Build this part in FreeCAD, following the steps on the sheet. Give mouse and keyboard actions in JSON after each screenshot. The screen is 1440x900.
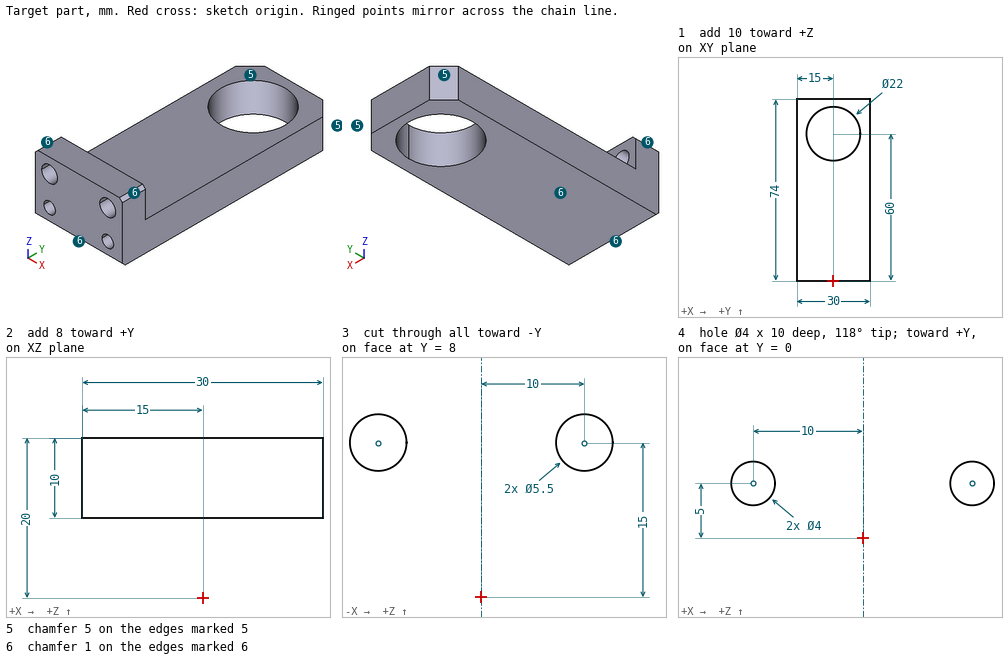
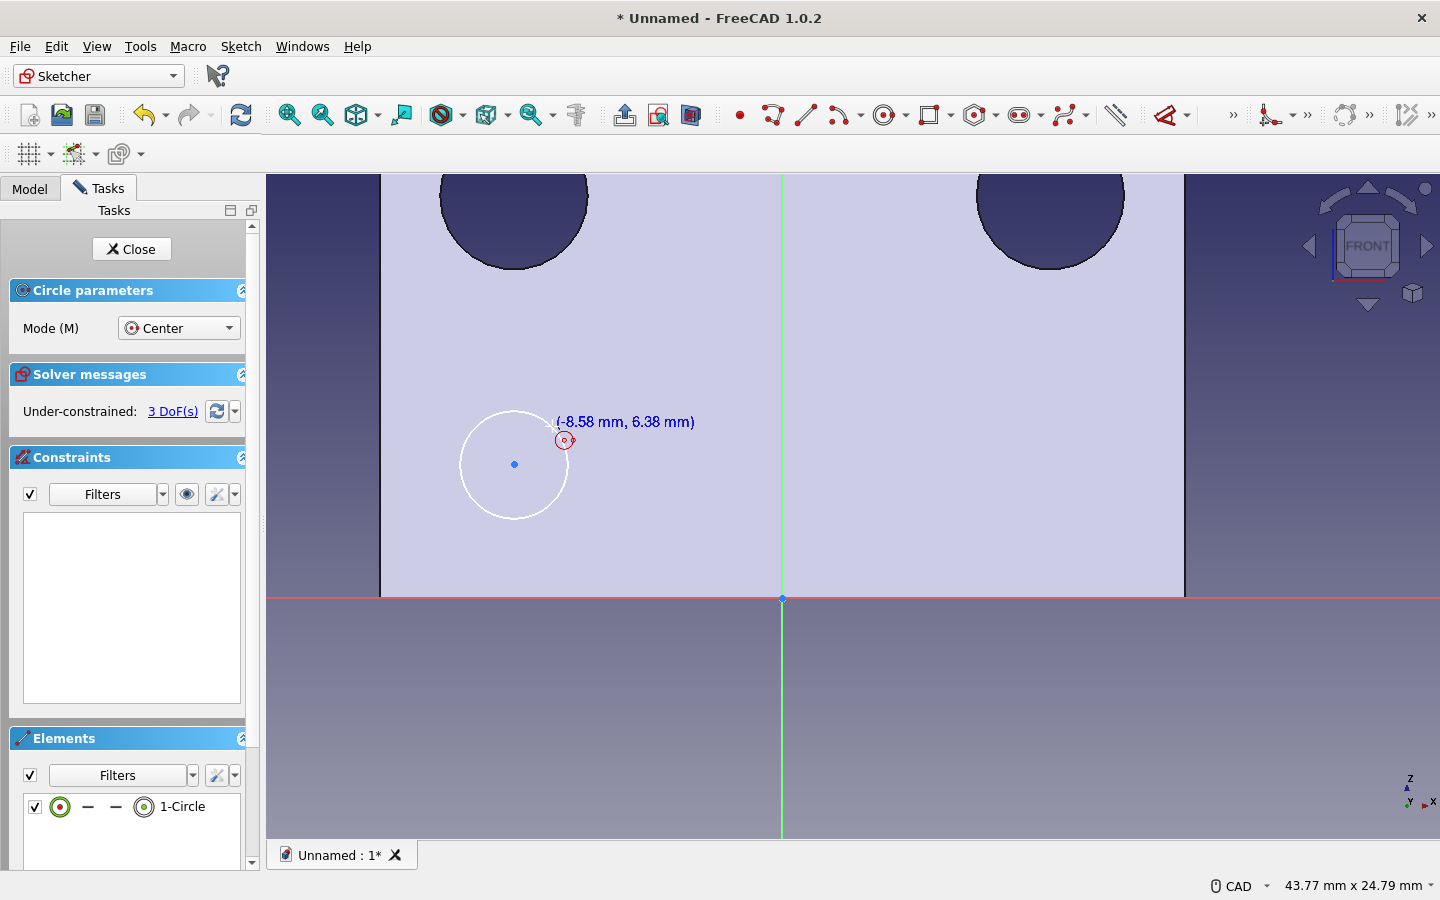
{"action": "left_click", "coordinate": [1050, 464]}
{"action": "left_click", "coordinate": [1088, 426]}
{"action": "key", "text": "Escape"}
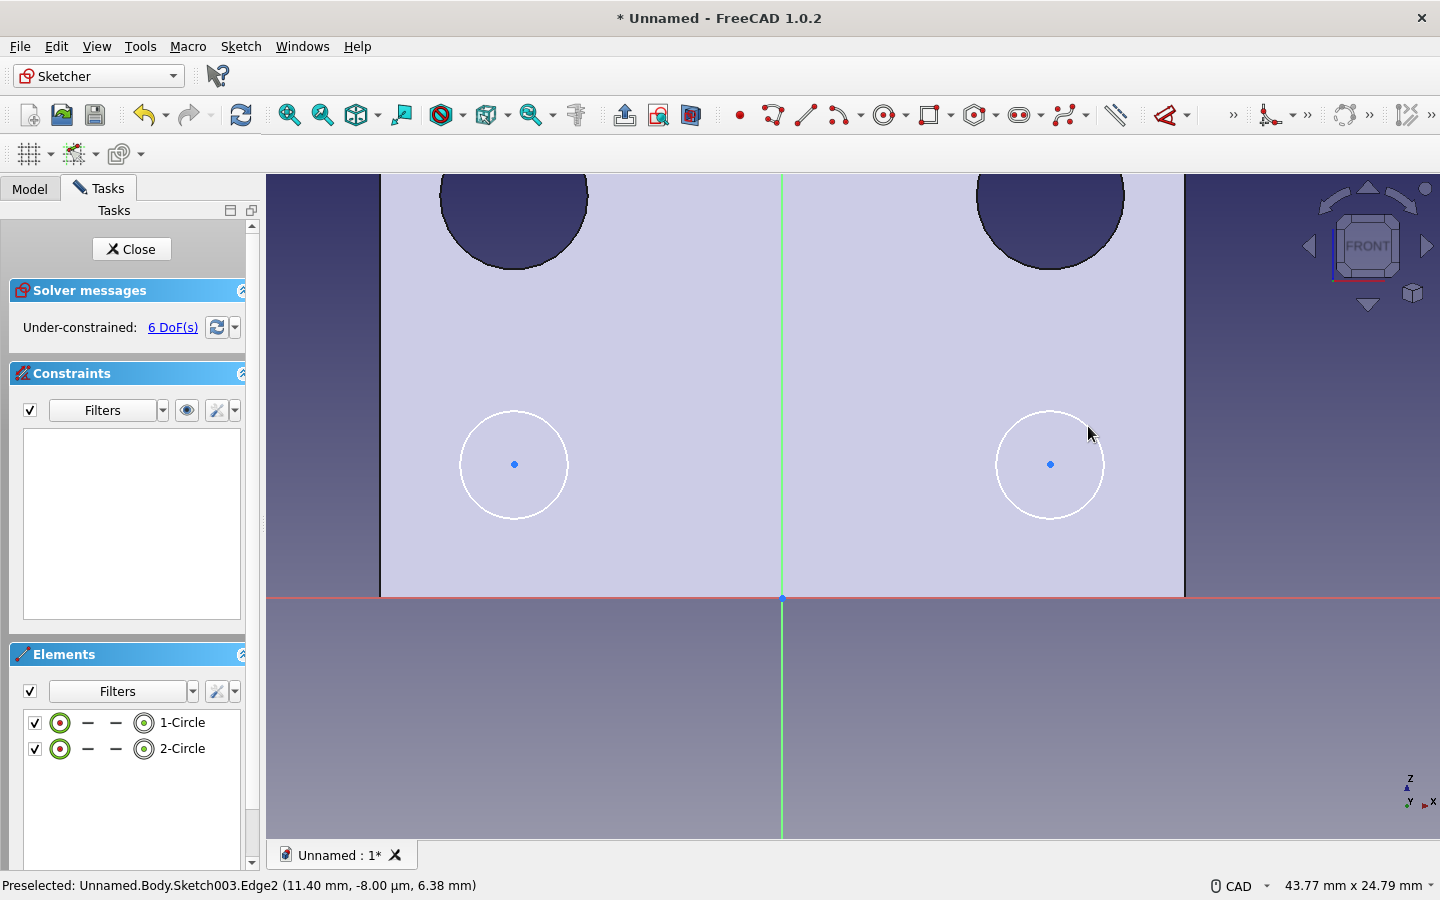
{"action": "left_click", "coordinate": [552, 427]}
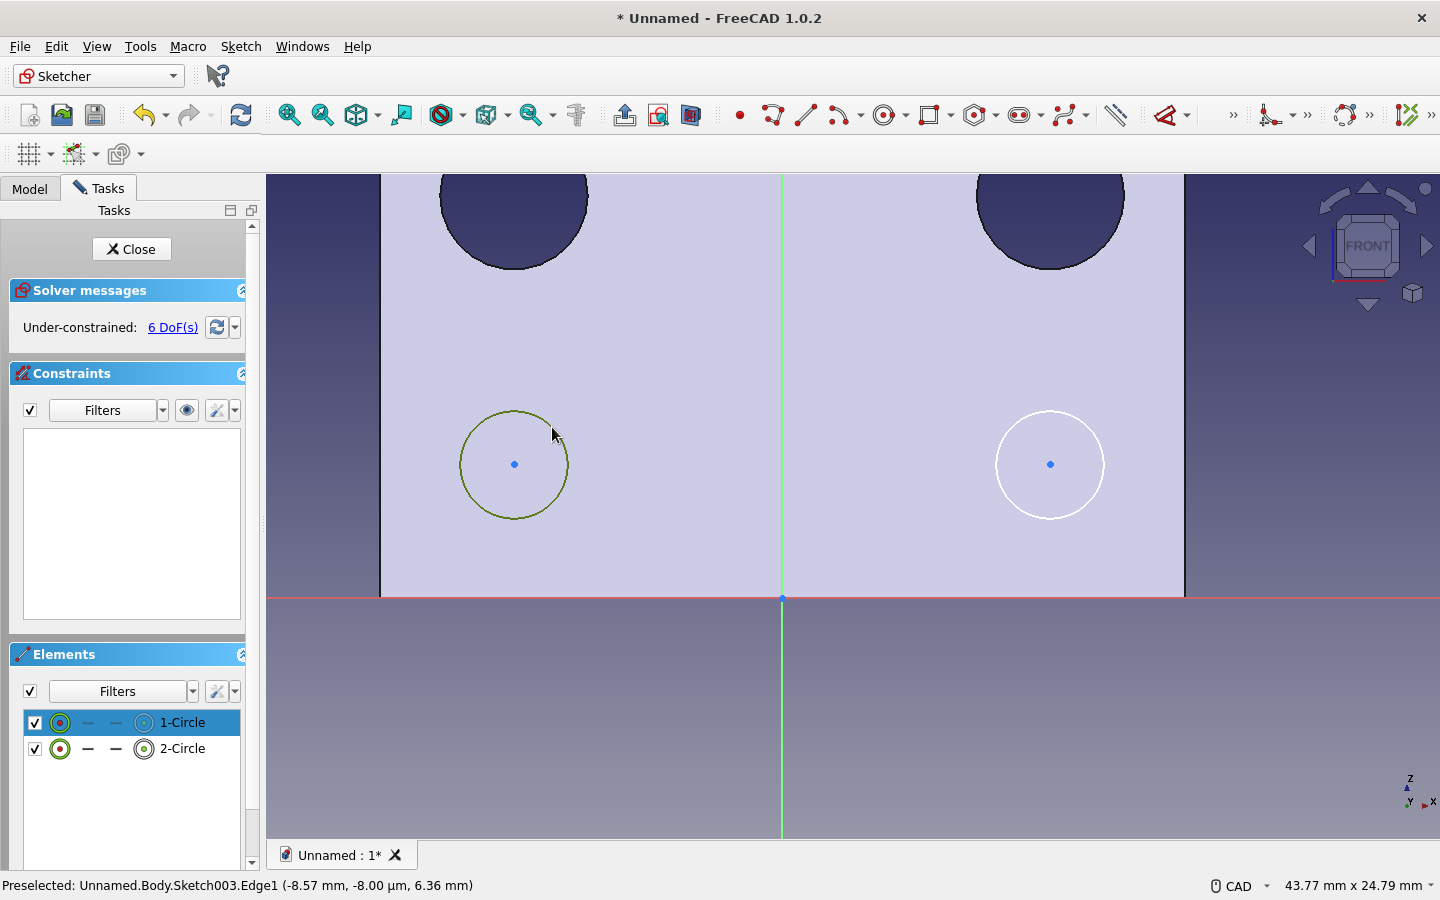
{"action": "left_click", "coordinate": [1088, 427]}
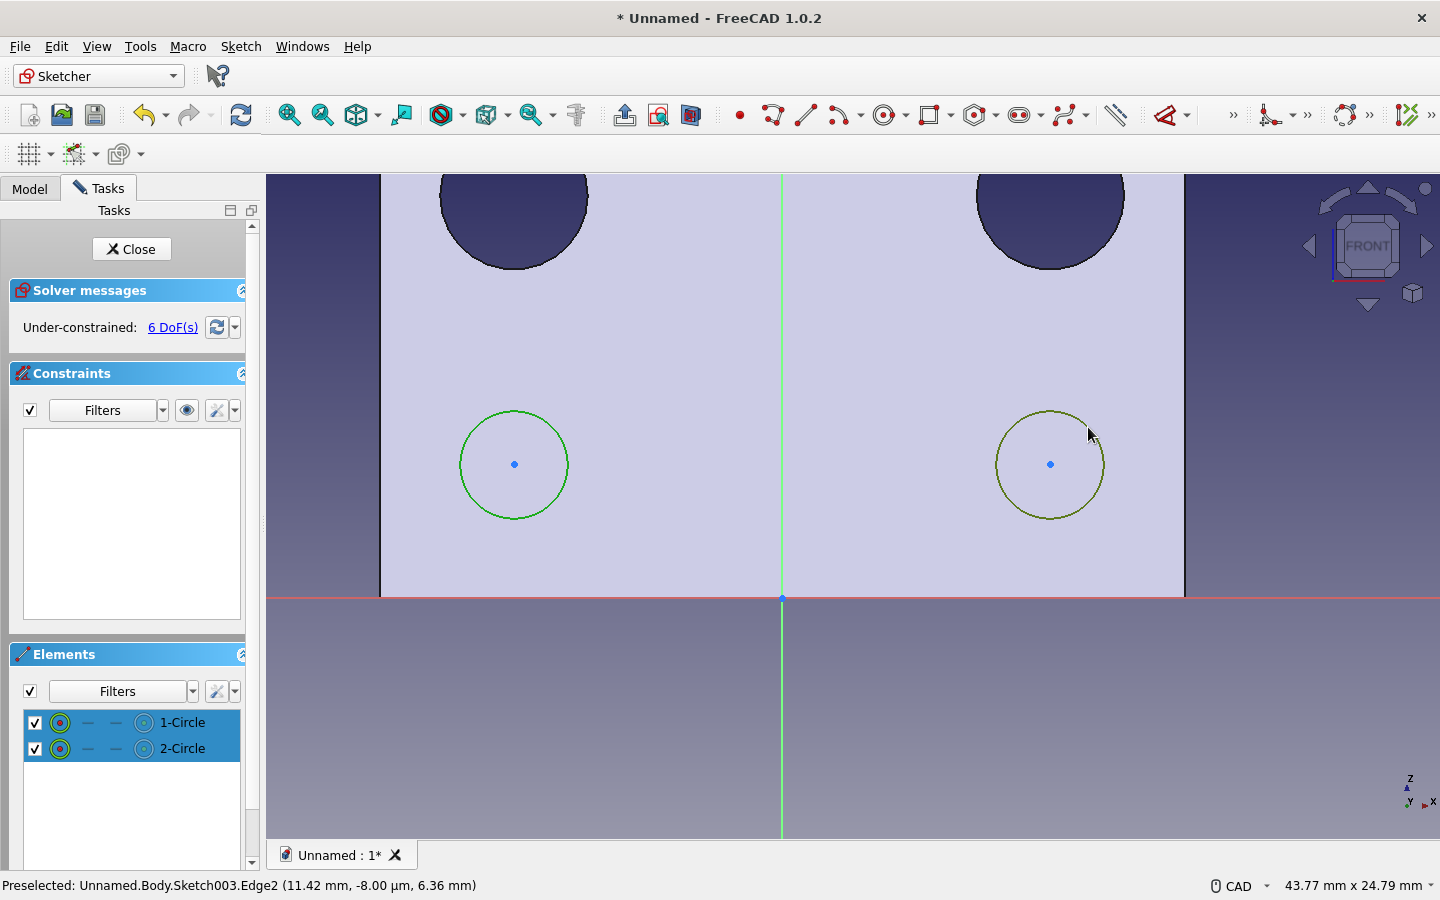
{"action": "key", "text": "e"}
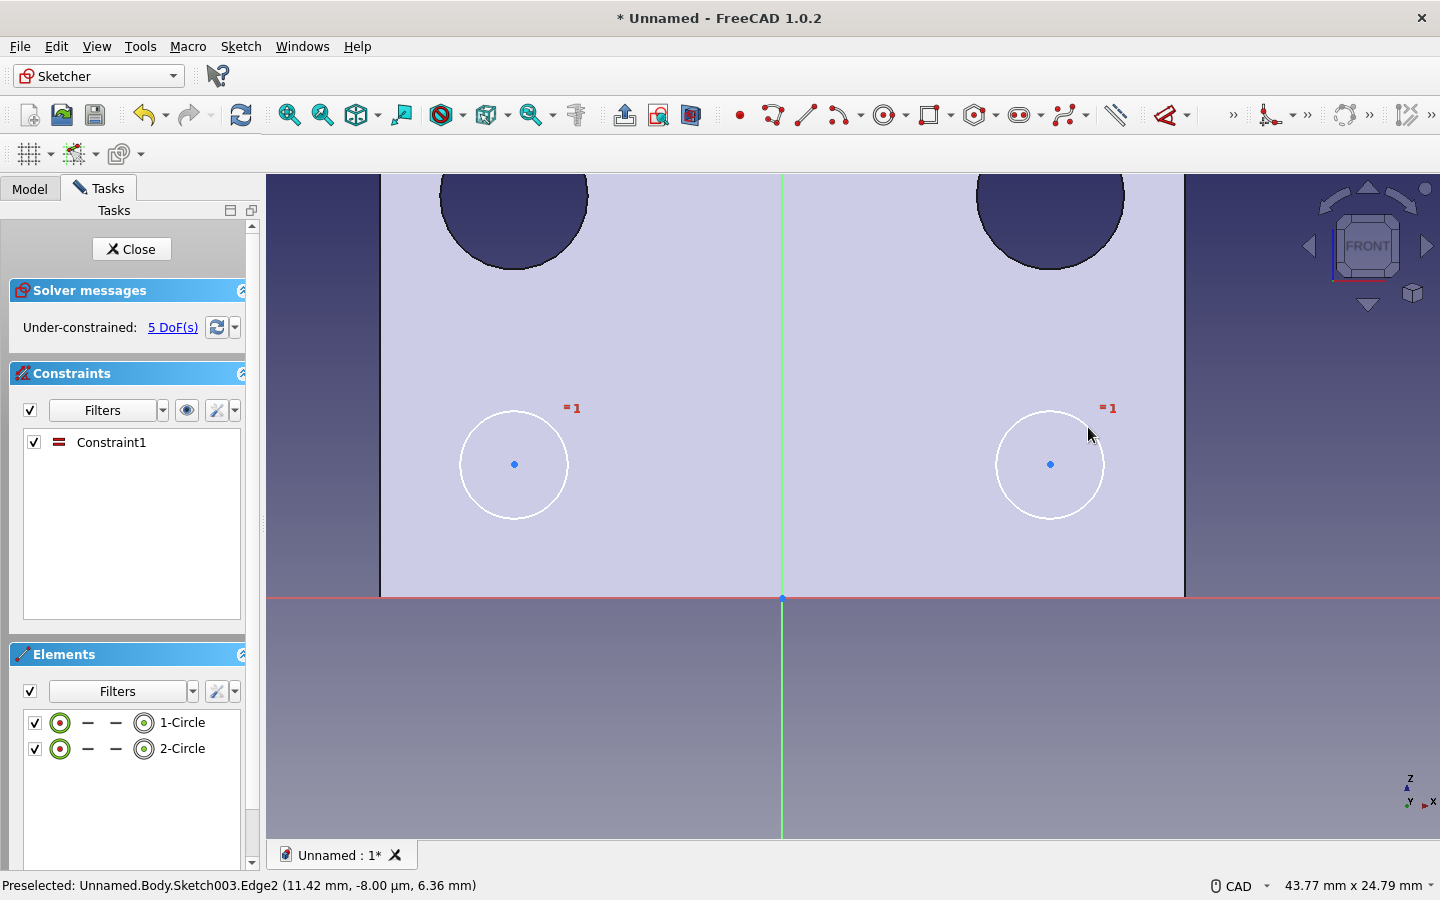
{"action": "left_click", "coordinate": [514, 465]}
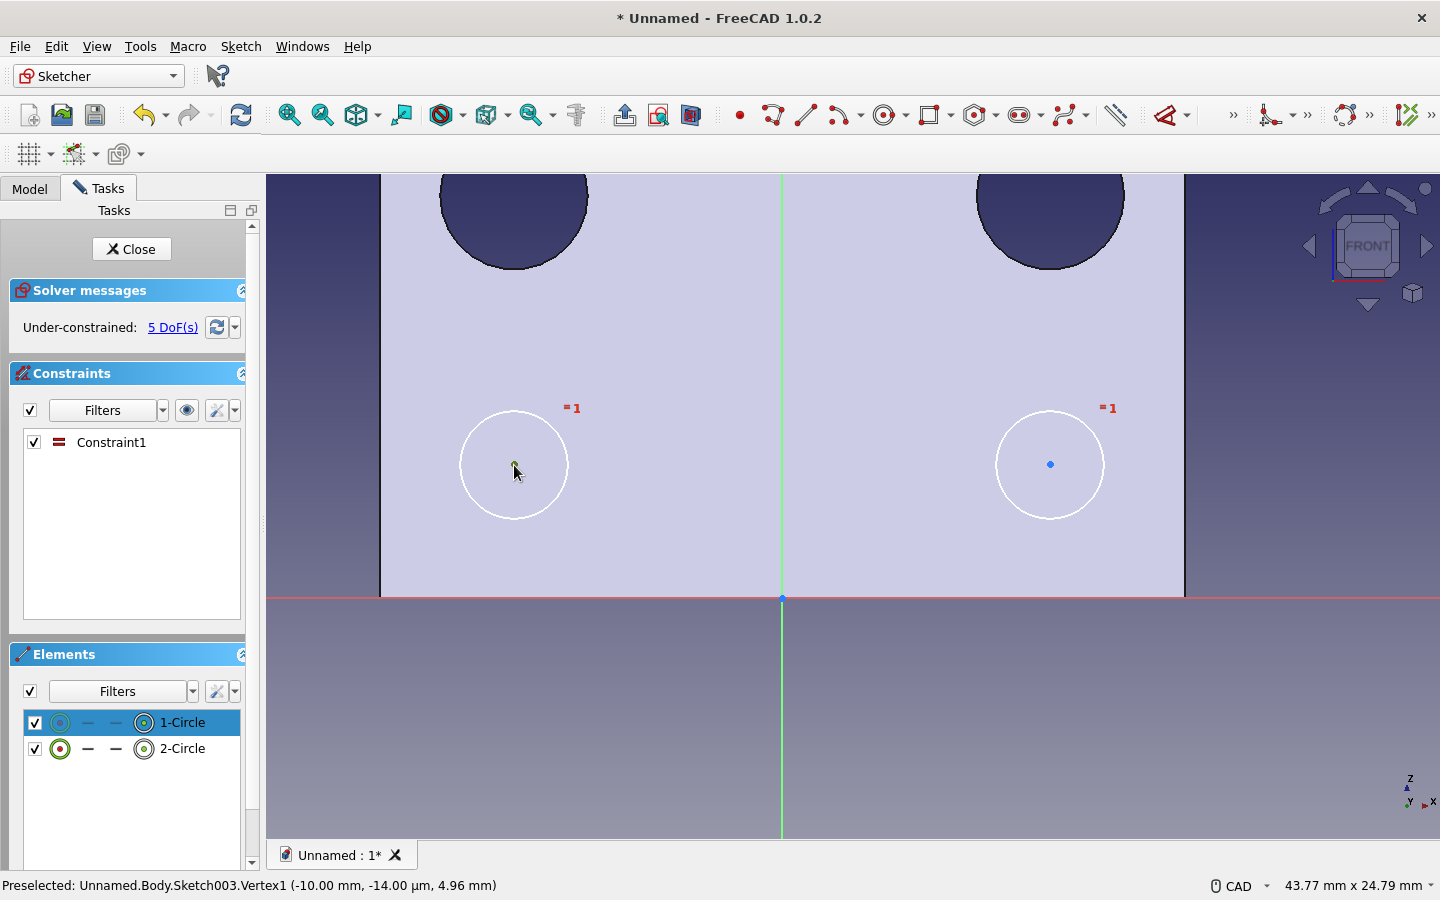
{"action": "left_click", "coordinate": [1050, 465]}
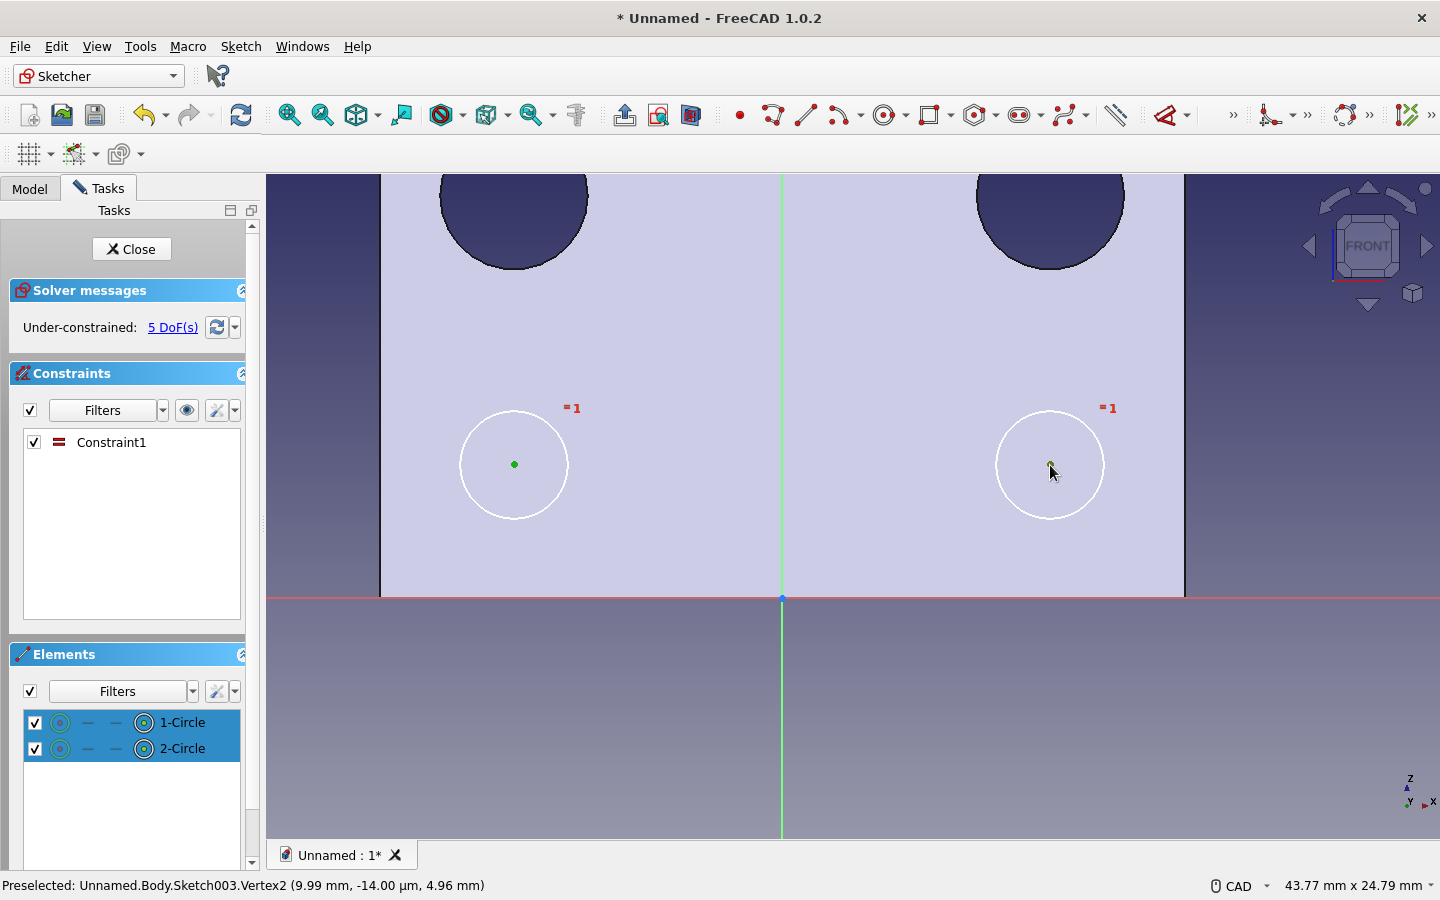
{"action": "left_click", "coordinate": [782, 768]}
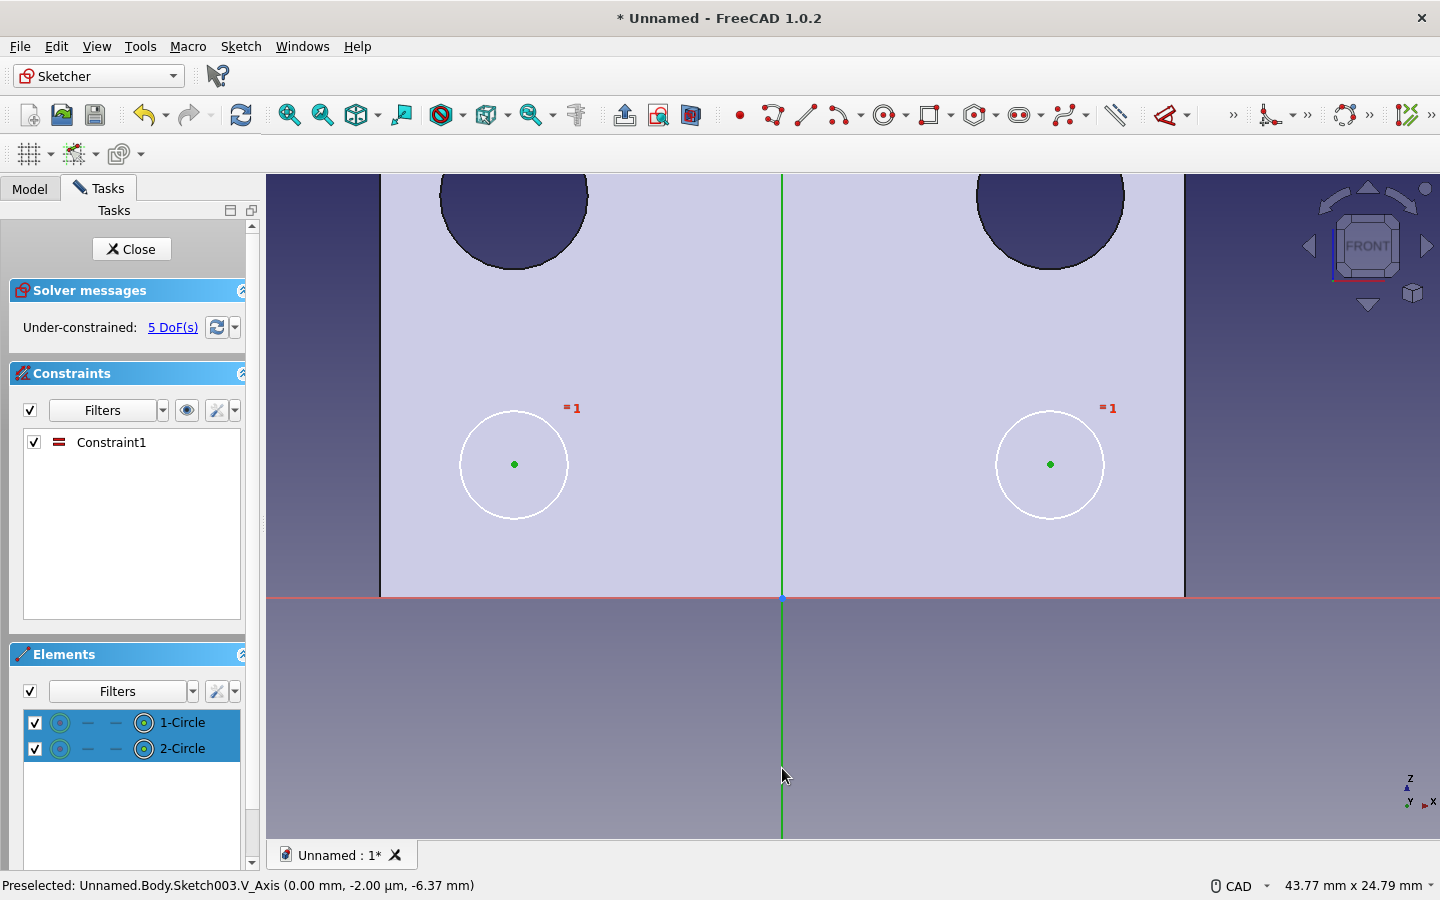
{"action": "key", "text": "s"}